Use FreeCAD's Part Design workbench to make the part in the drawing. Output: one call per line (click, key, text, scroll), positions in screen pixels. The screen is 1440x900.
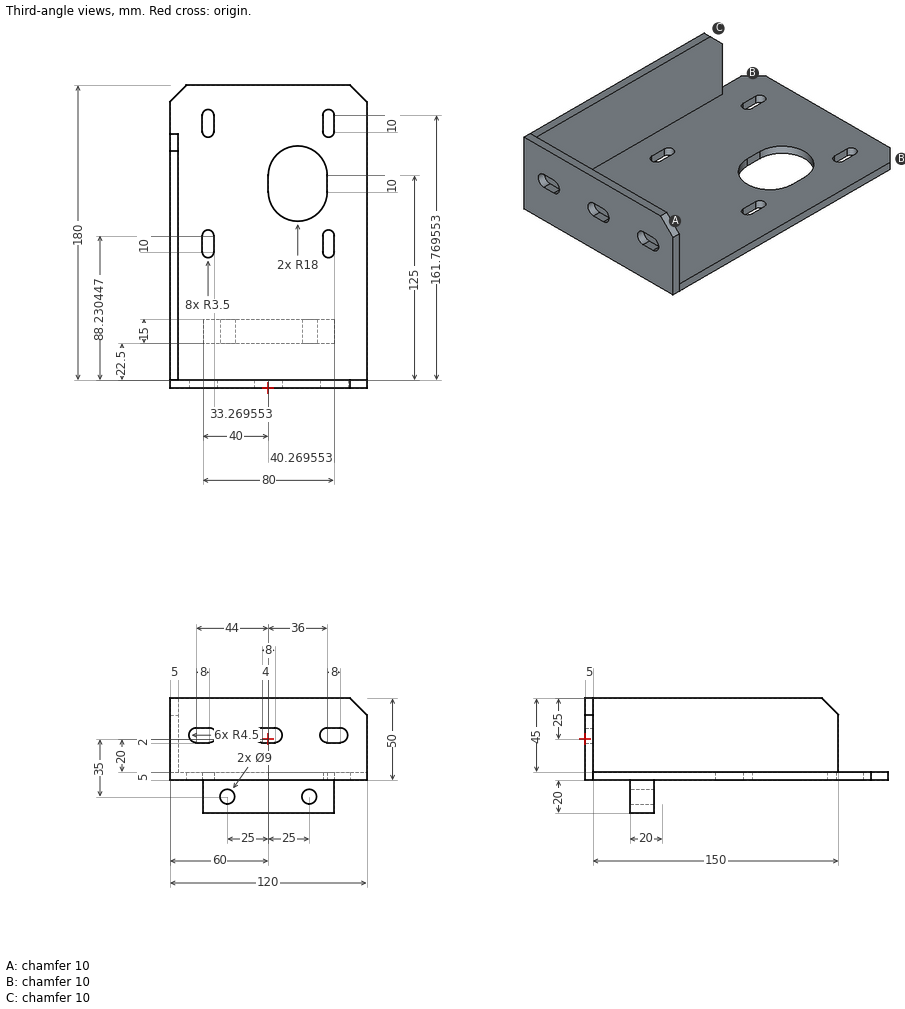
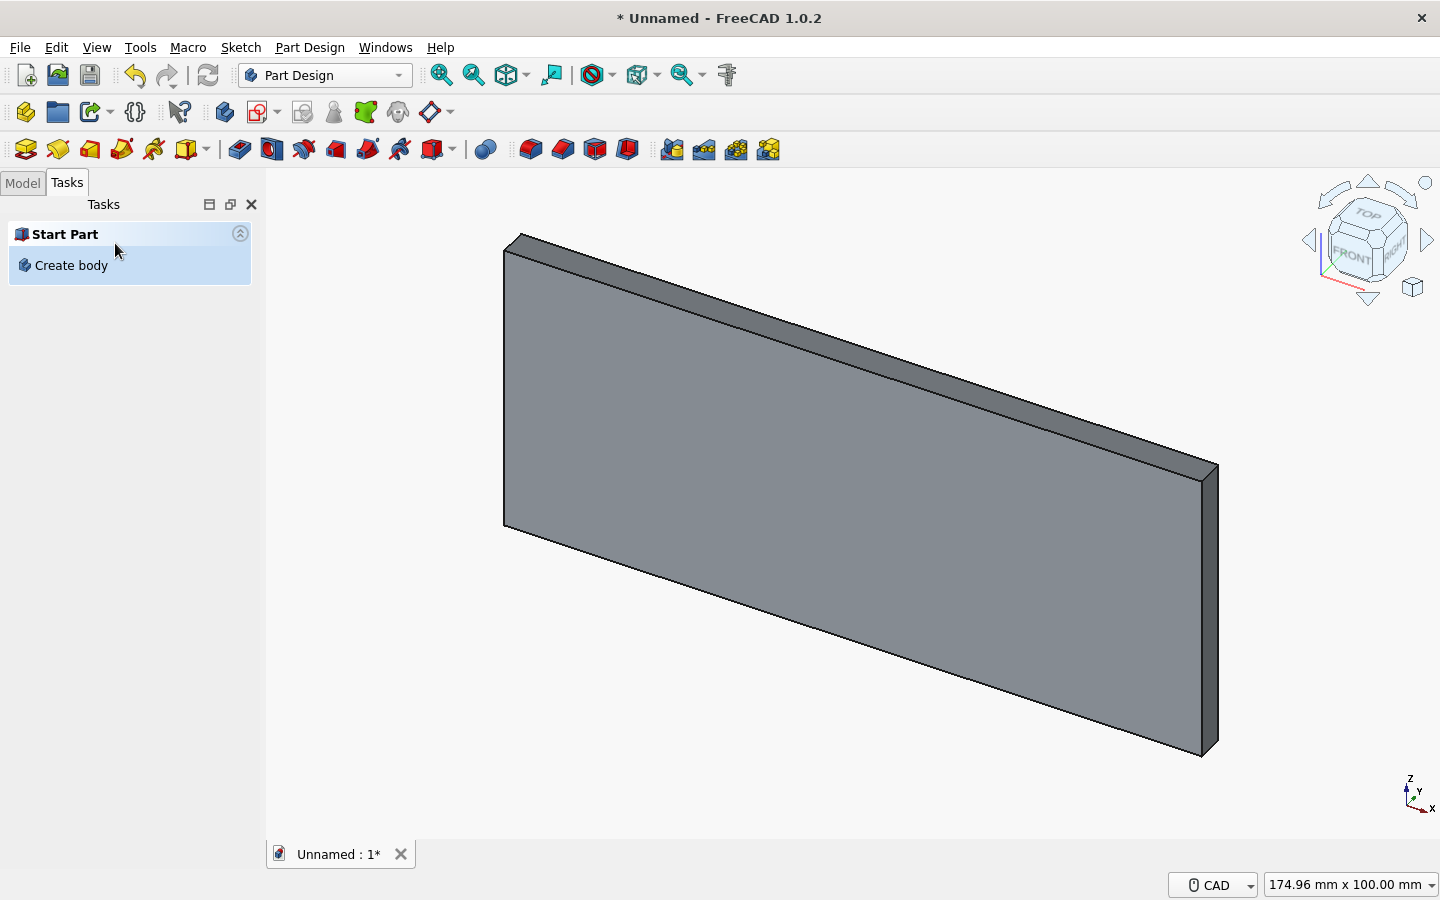
key(4)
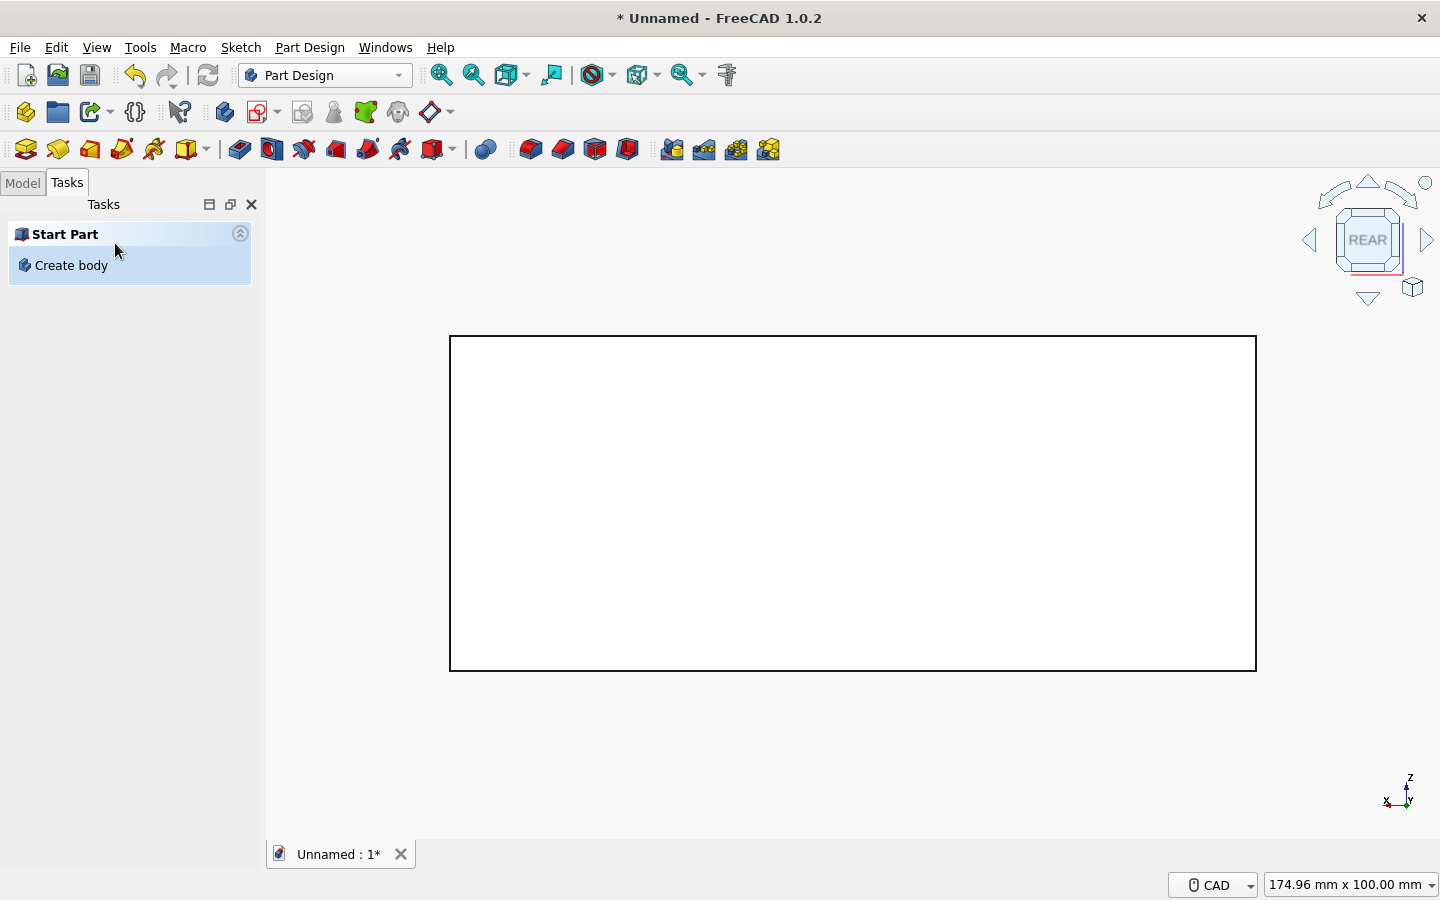
click(623, 502)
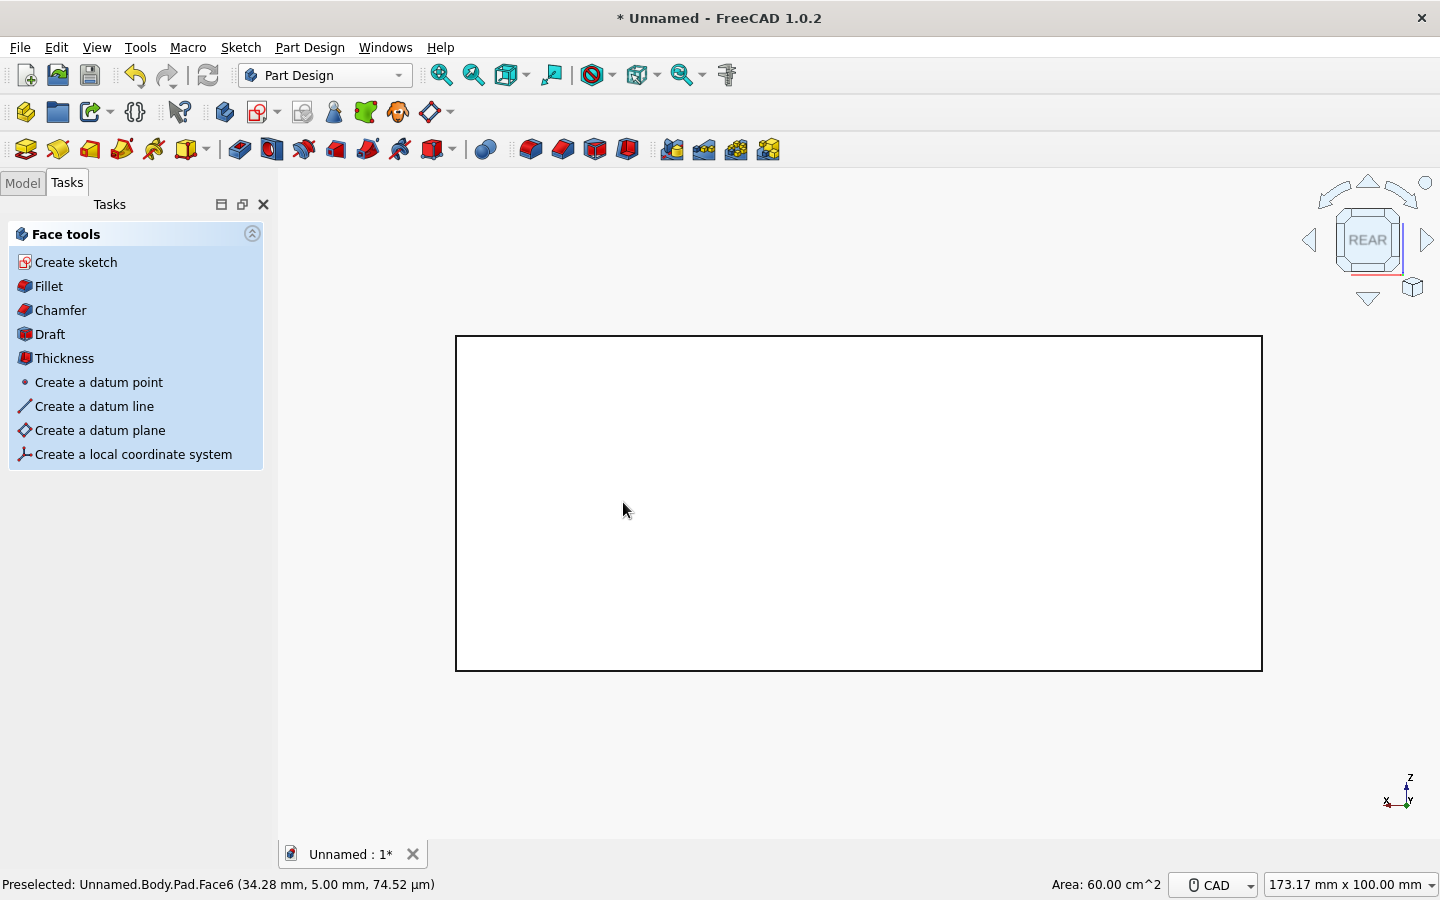
click(258, 112)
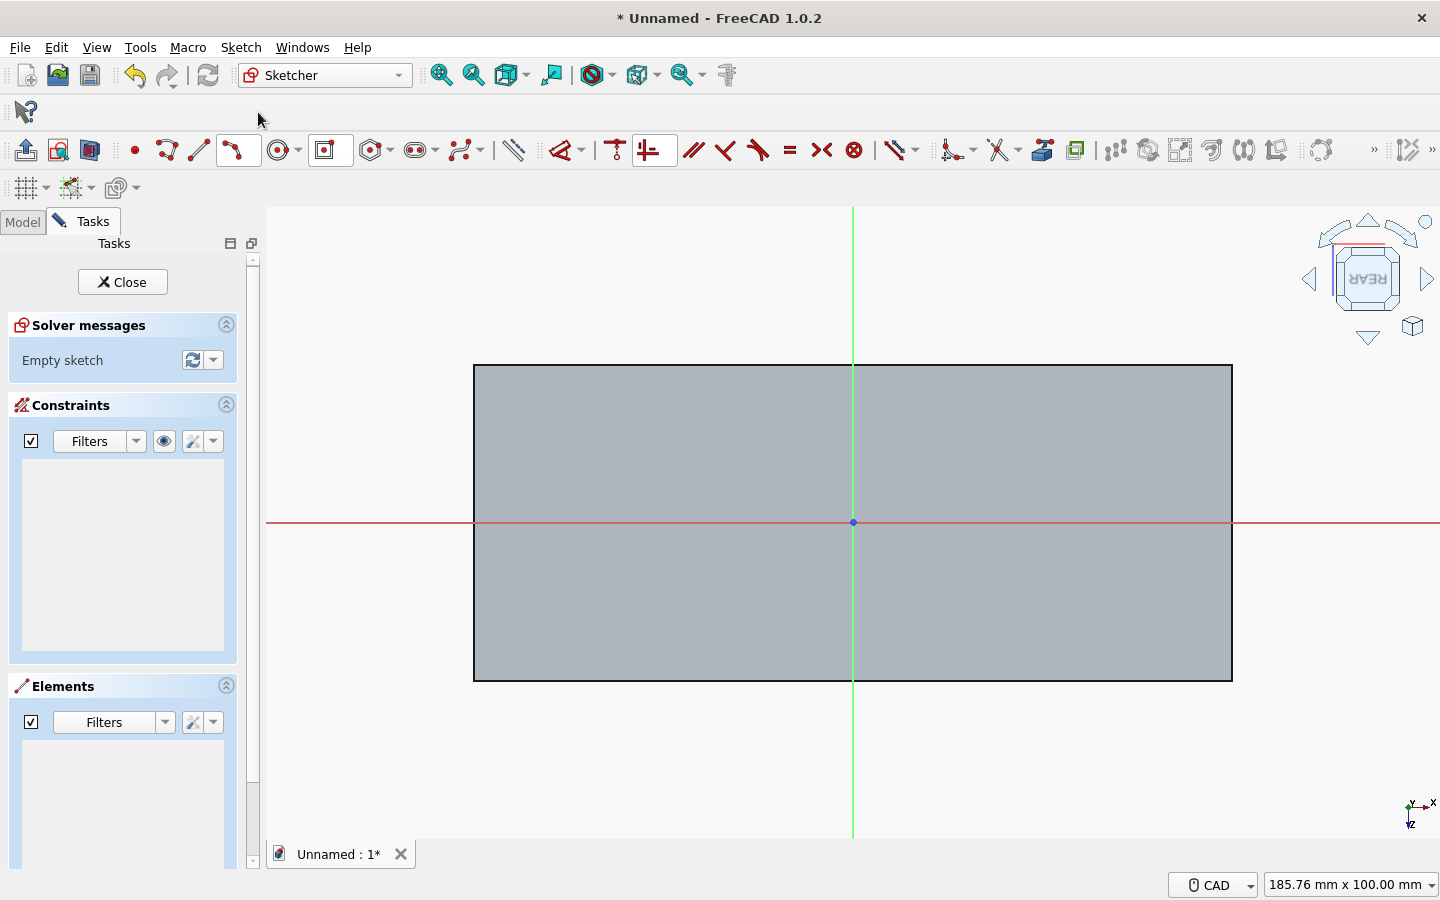
key(g)
key(s)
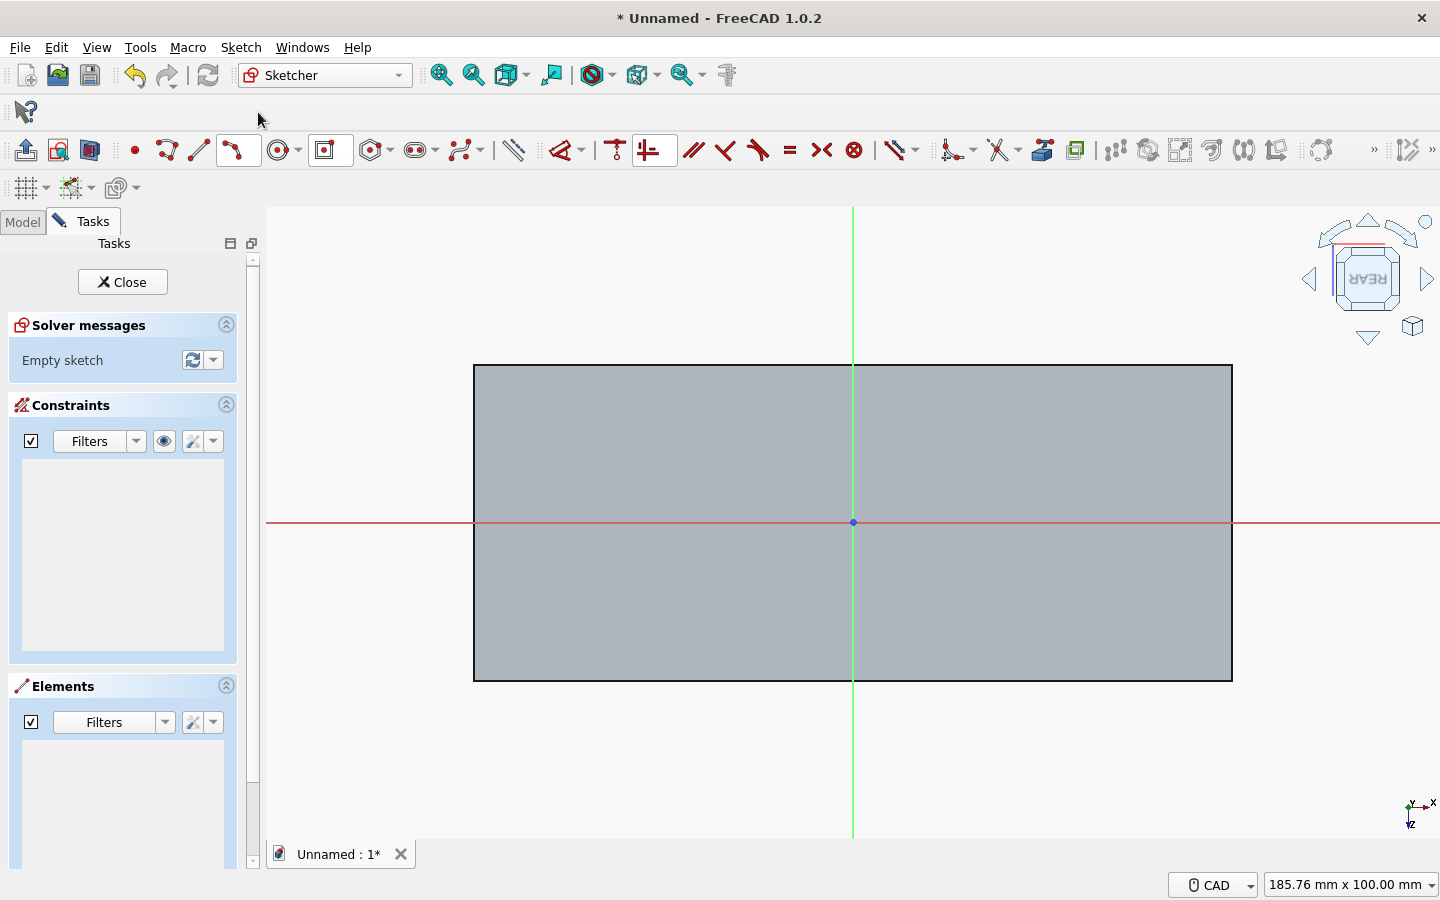
click(575, 539)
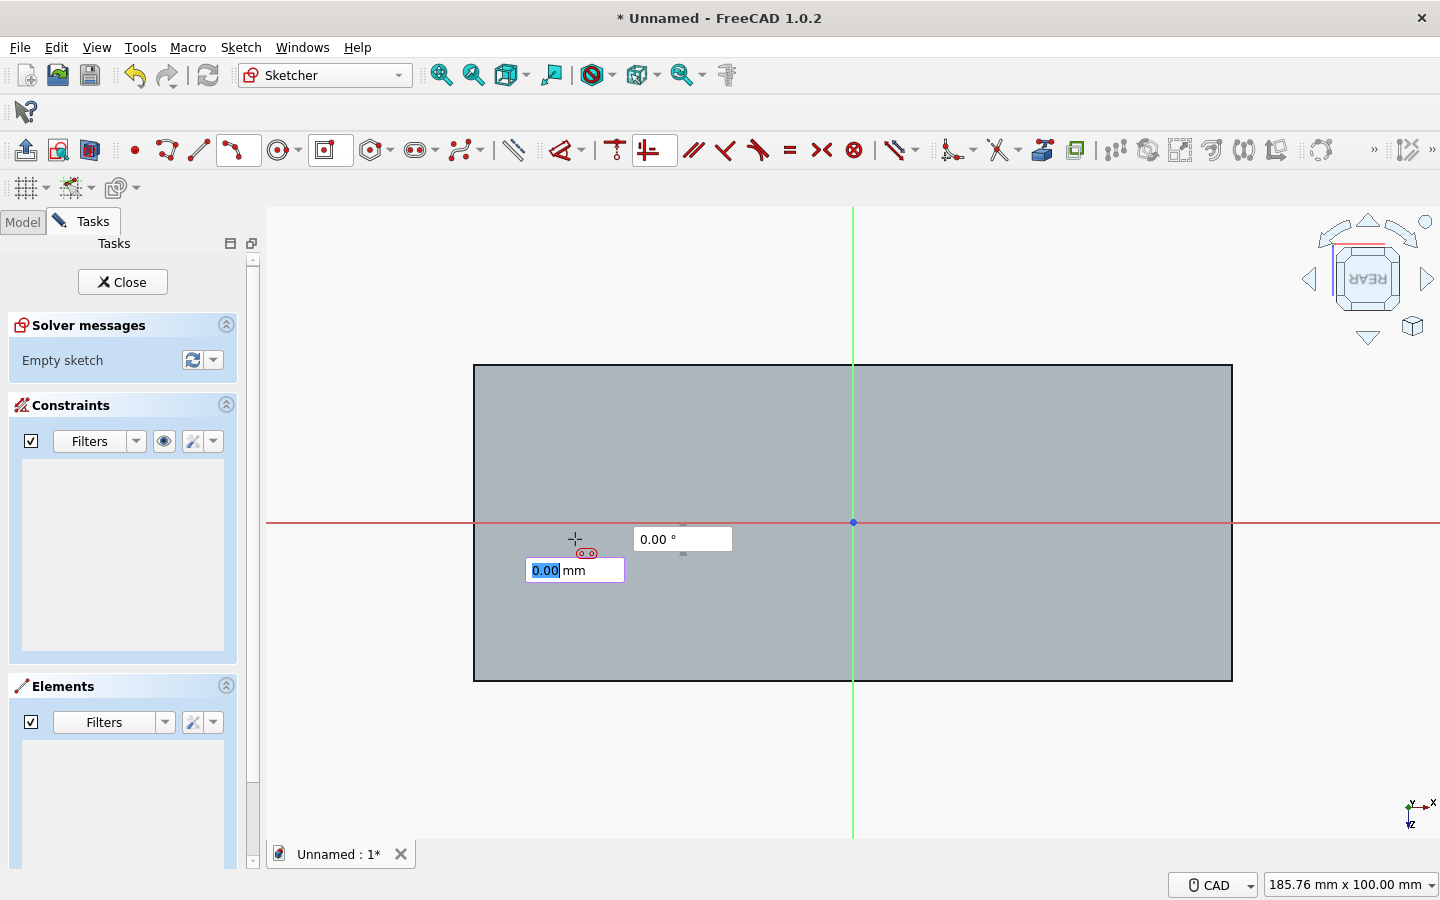
click(625, 539)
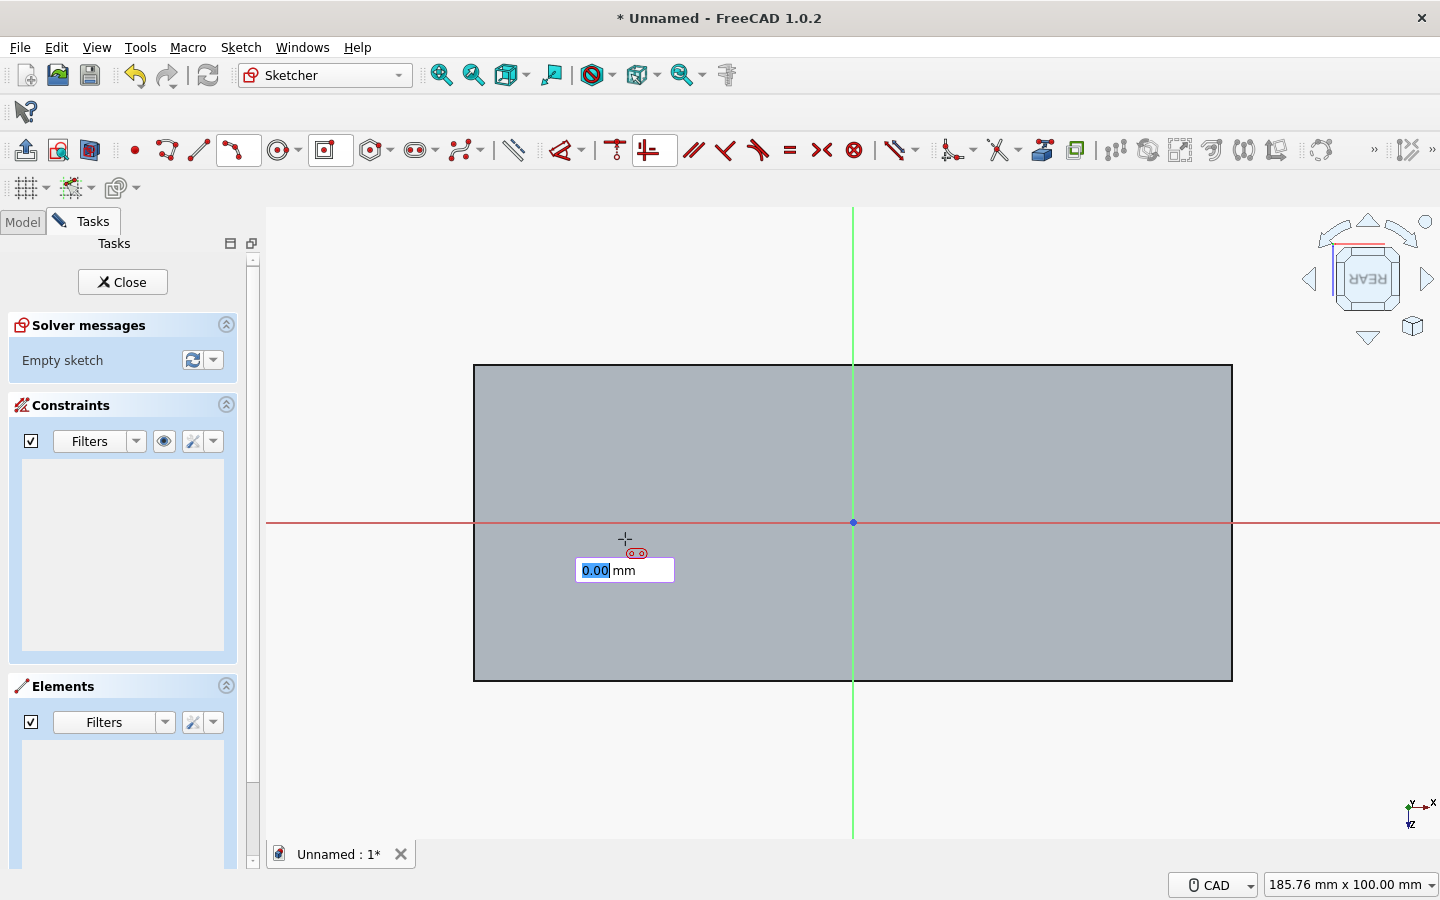
click(600, 567)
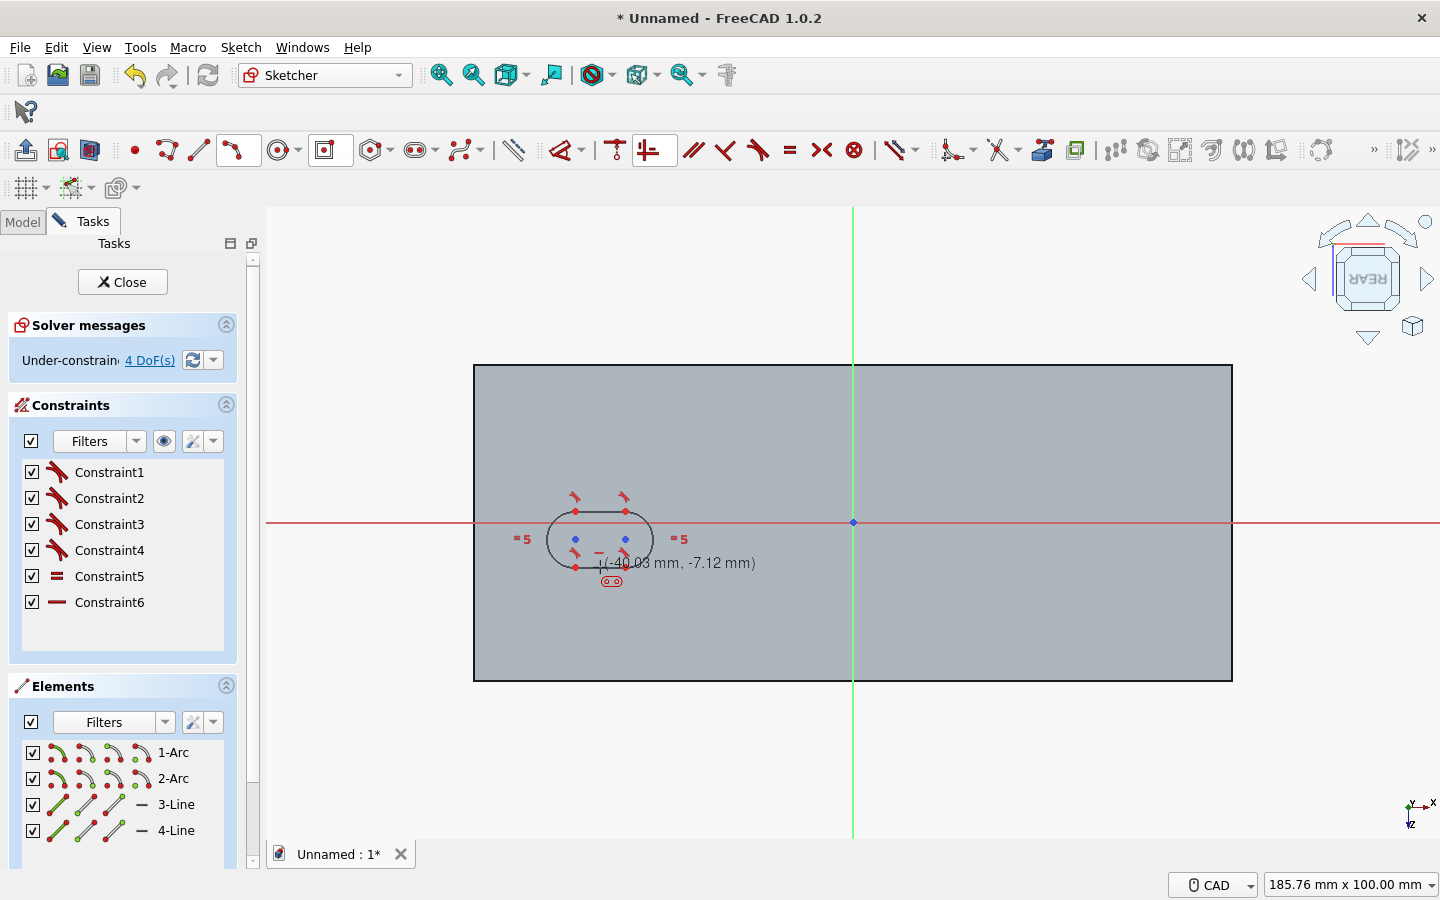
click(828, 539)